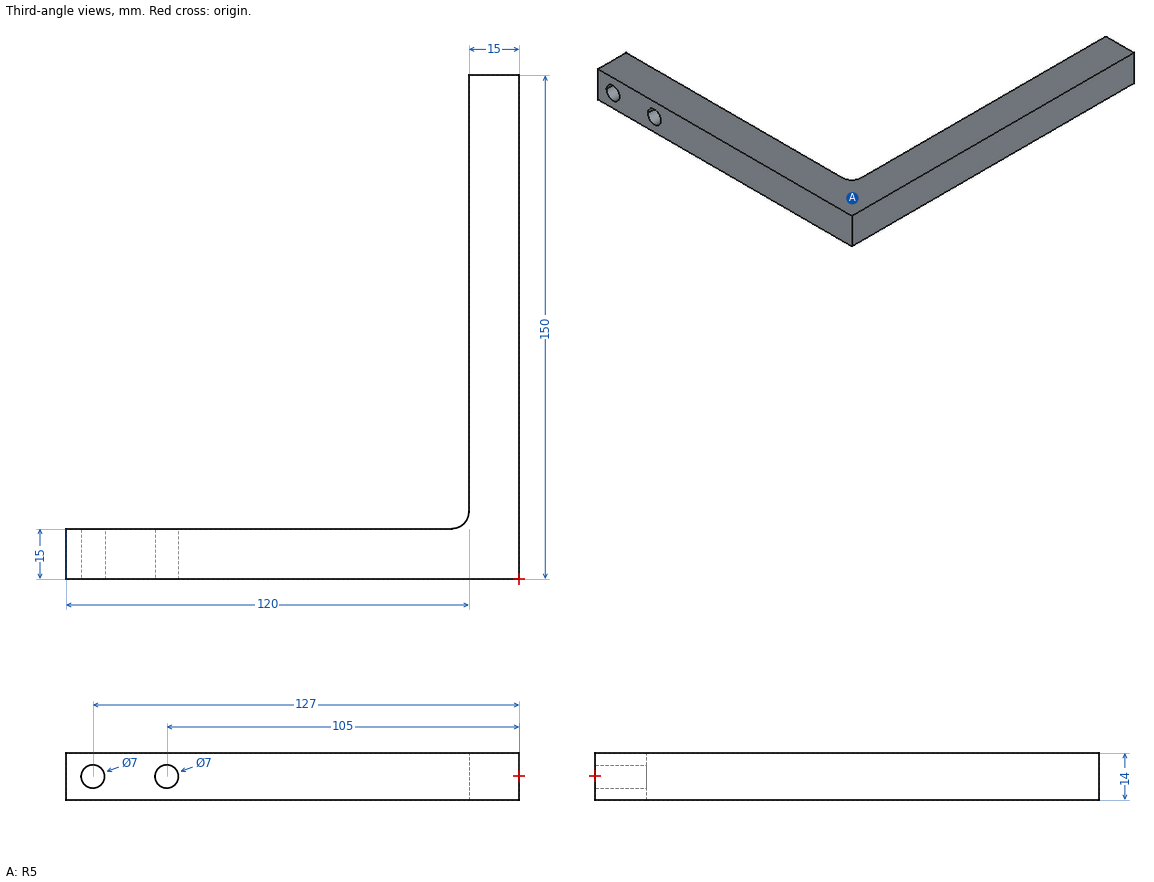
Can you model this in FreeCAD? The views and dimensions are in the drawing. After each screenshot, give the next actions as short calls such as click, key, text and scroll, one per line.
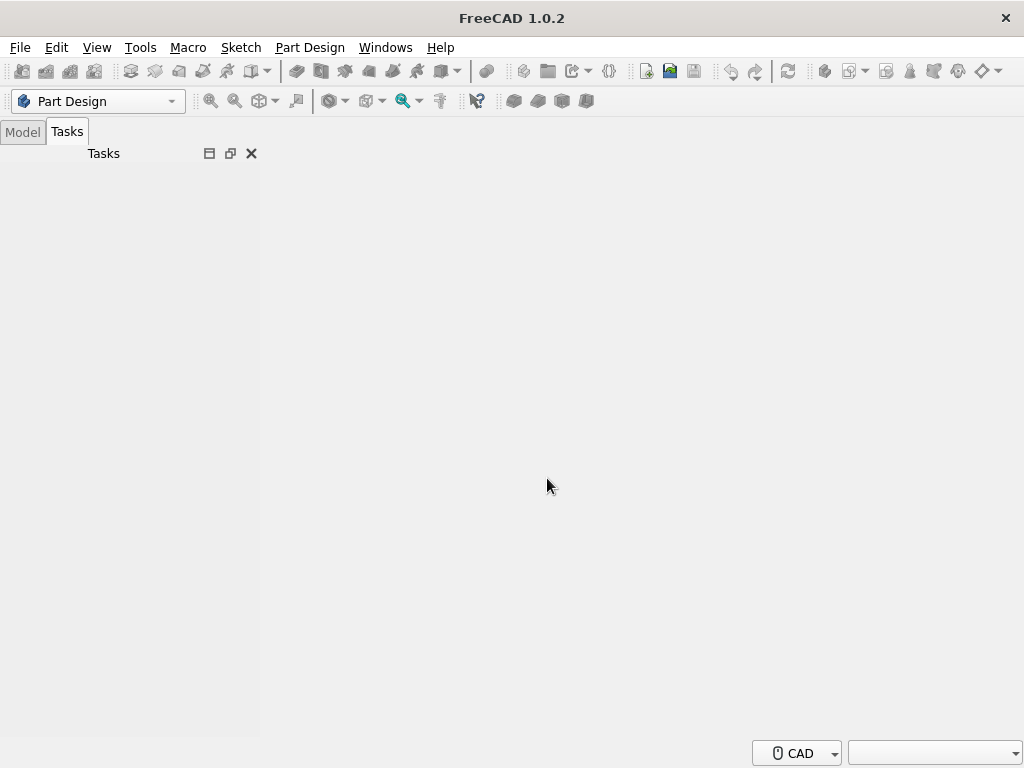
click(646, 72)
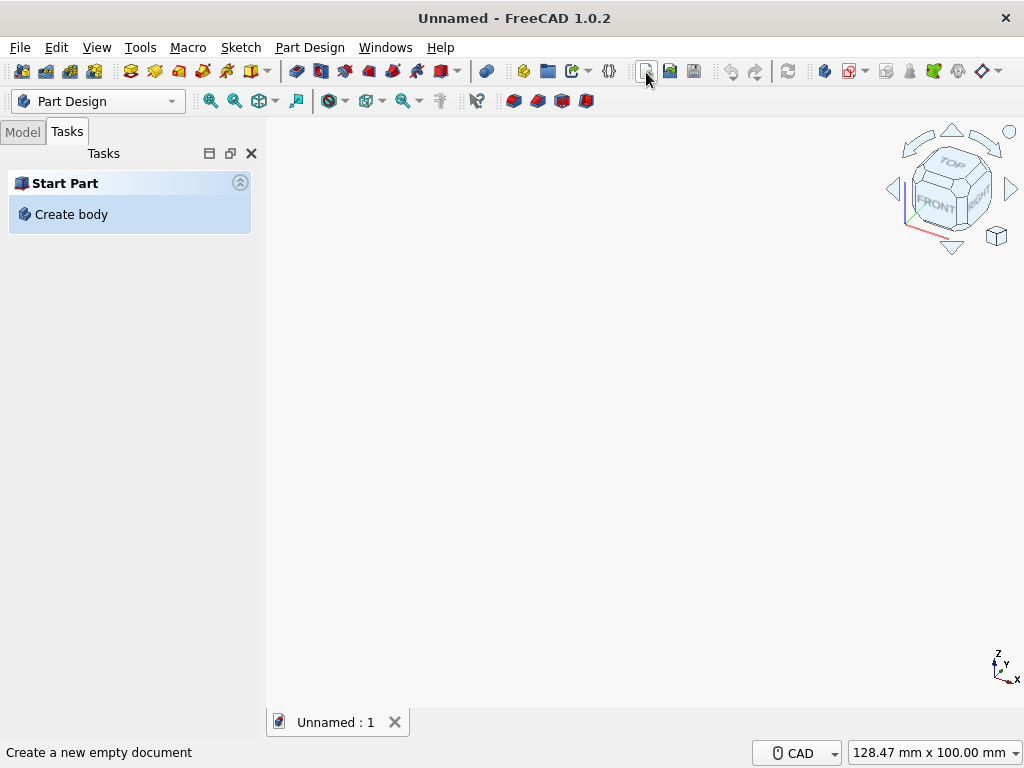
click(850, 72)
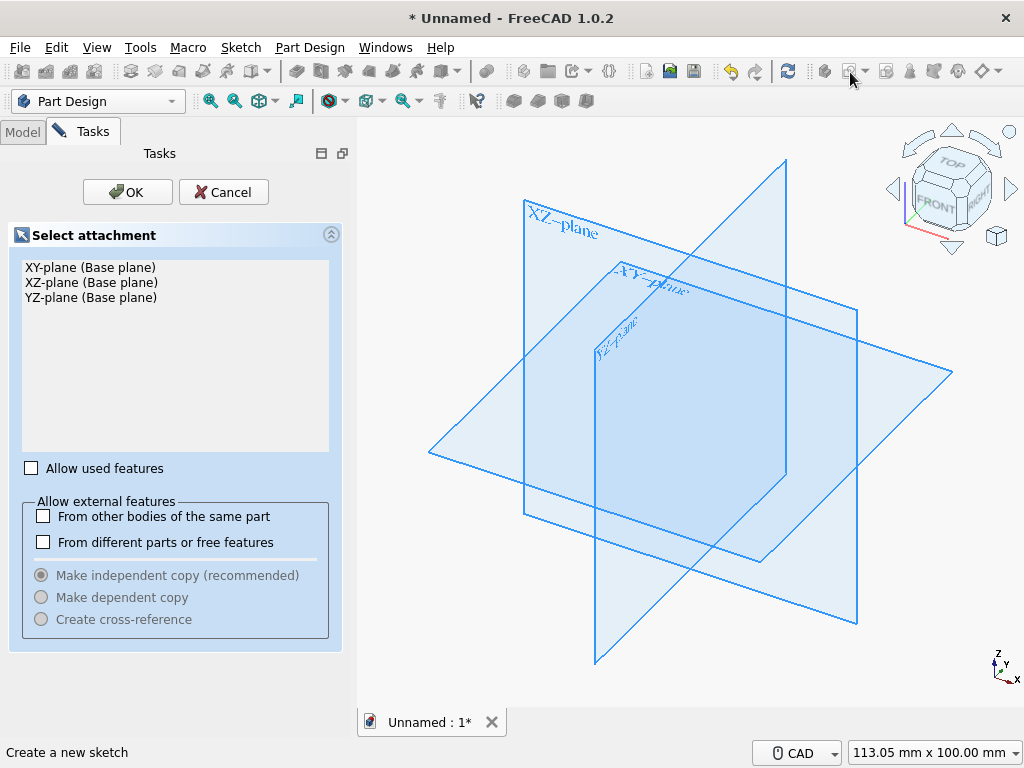
click(82, 268)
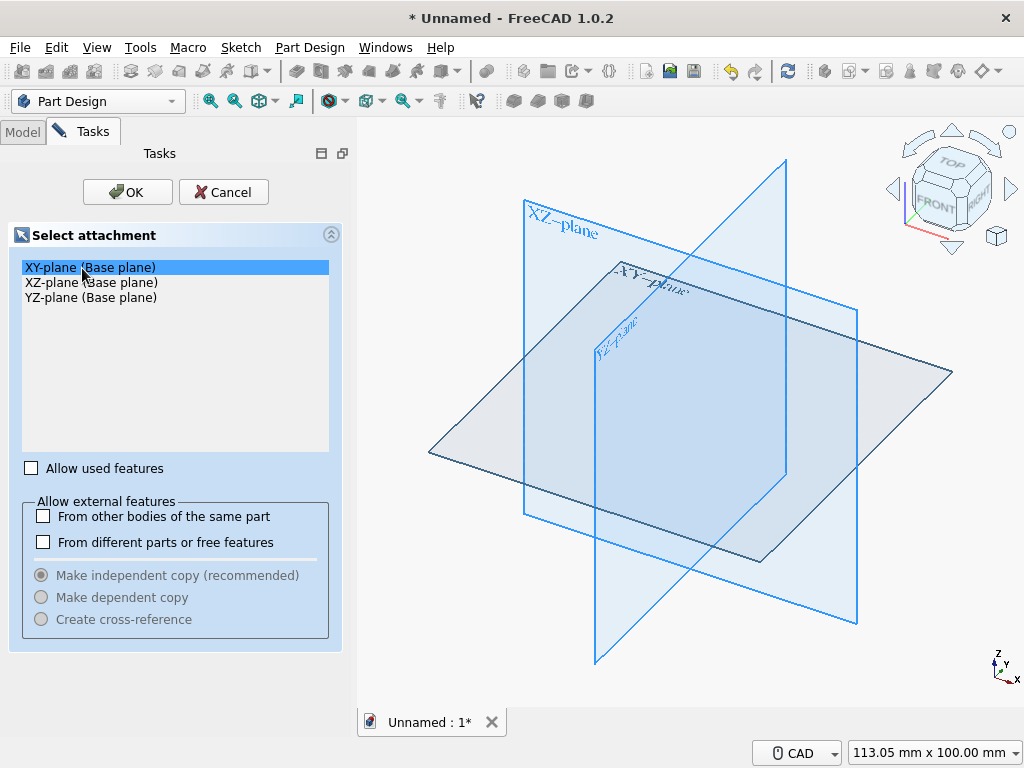
click(128, 192)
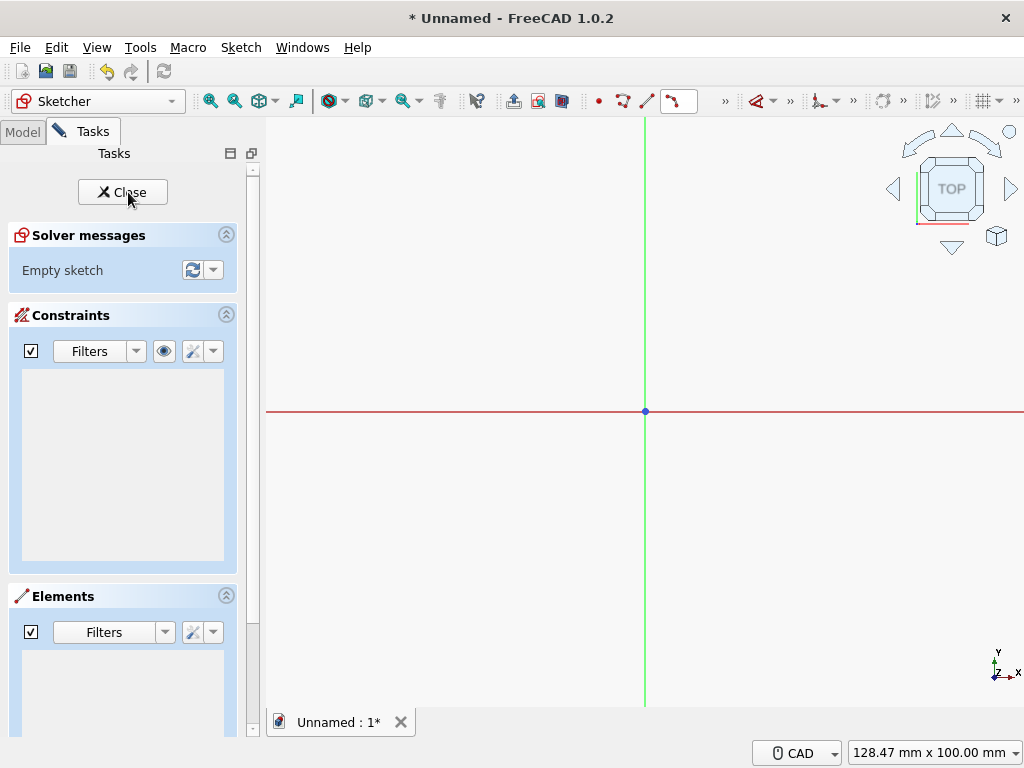
scroll(768, 670, down, 5)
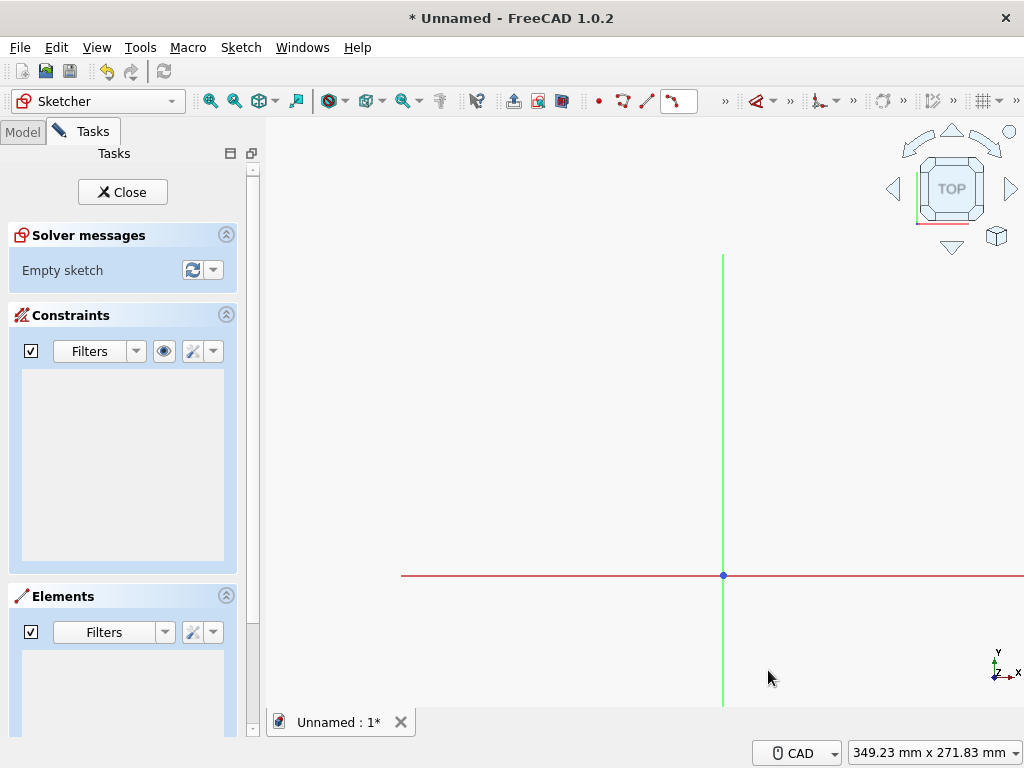
click(624, 102)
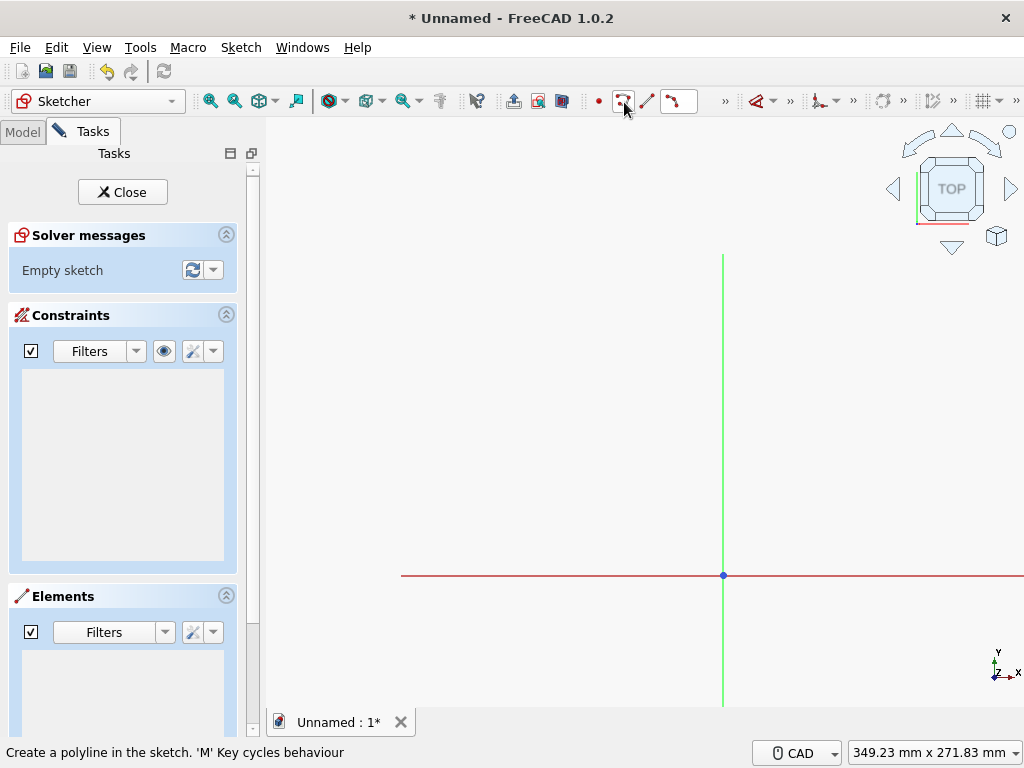
click(723, 576)
click(714, 250)
click(691, 250)
click(691, 543)
click(430, 543)
click(430, 567)
click(723, 576)
key(Escape)
key(Escape)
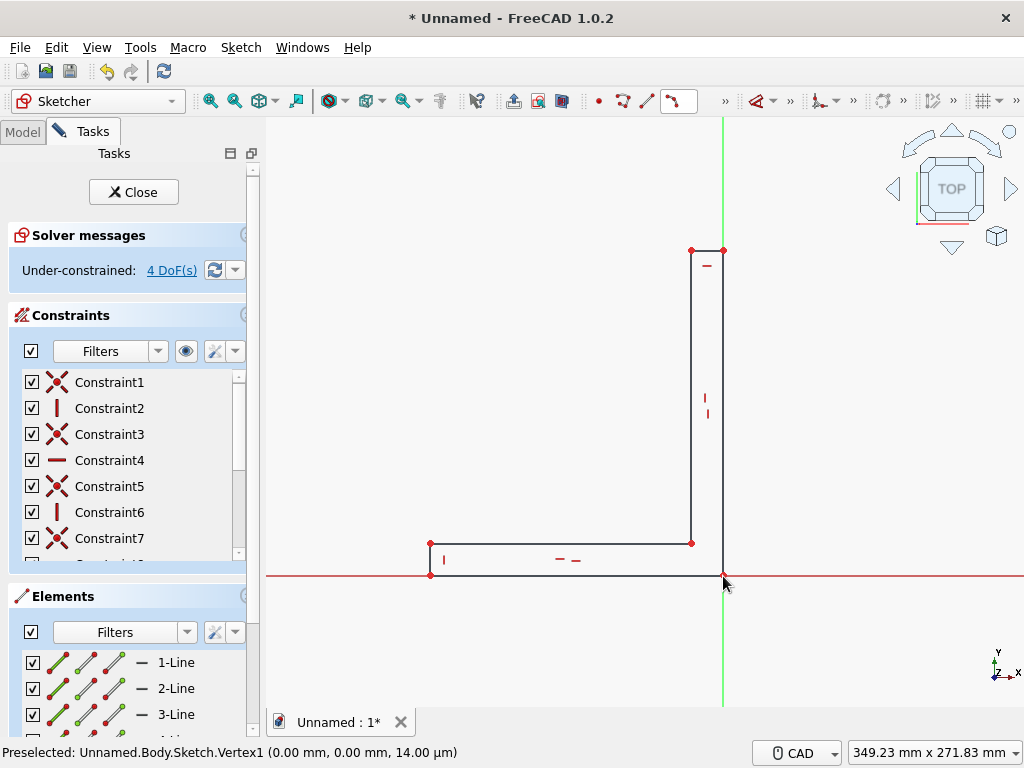
key(d)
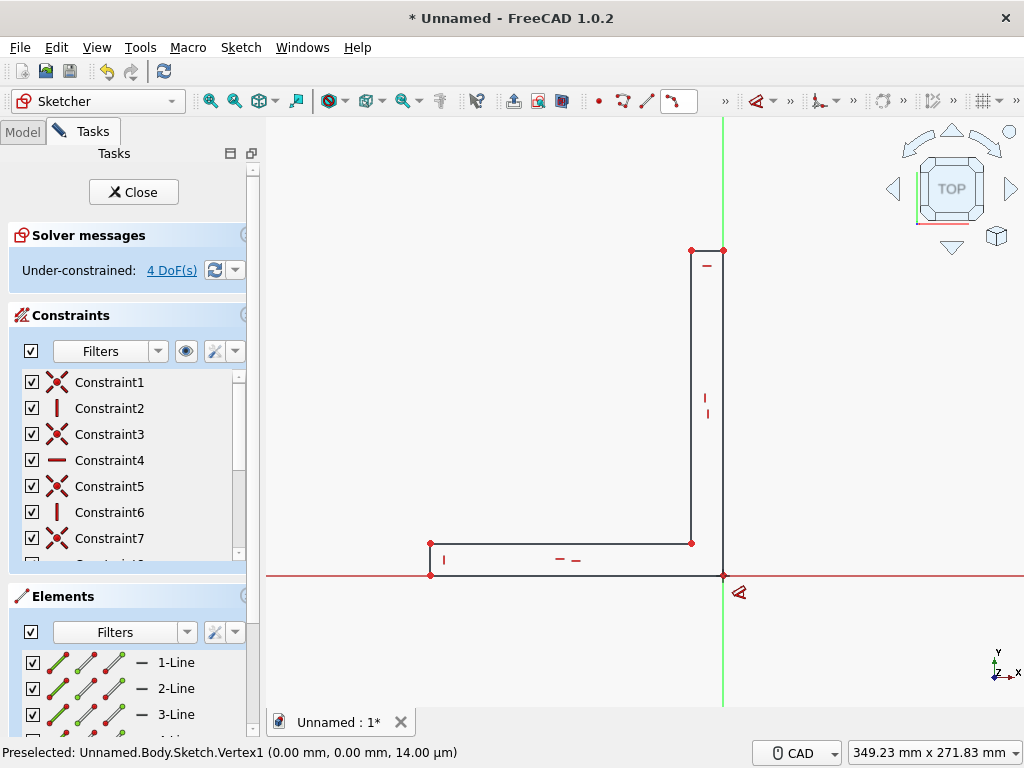
scroll(714, 251, up, 2)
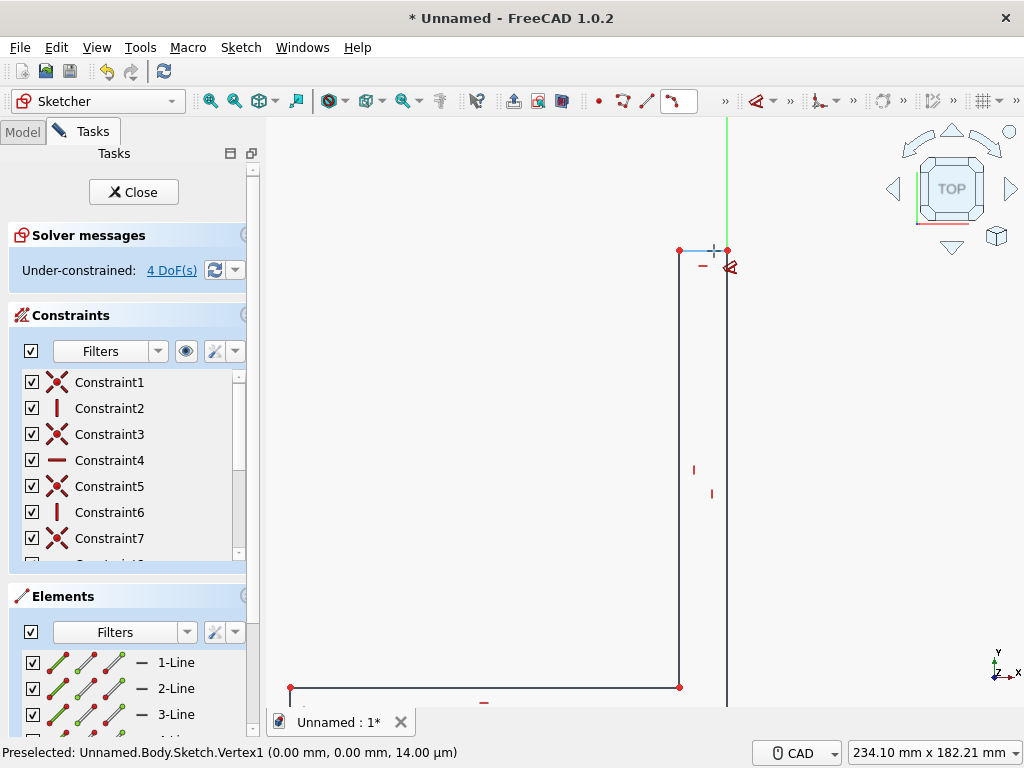
click(713, 251)
click(703, 217)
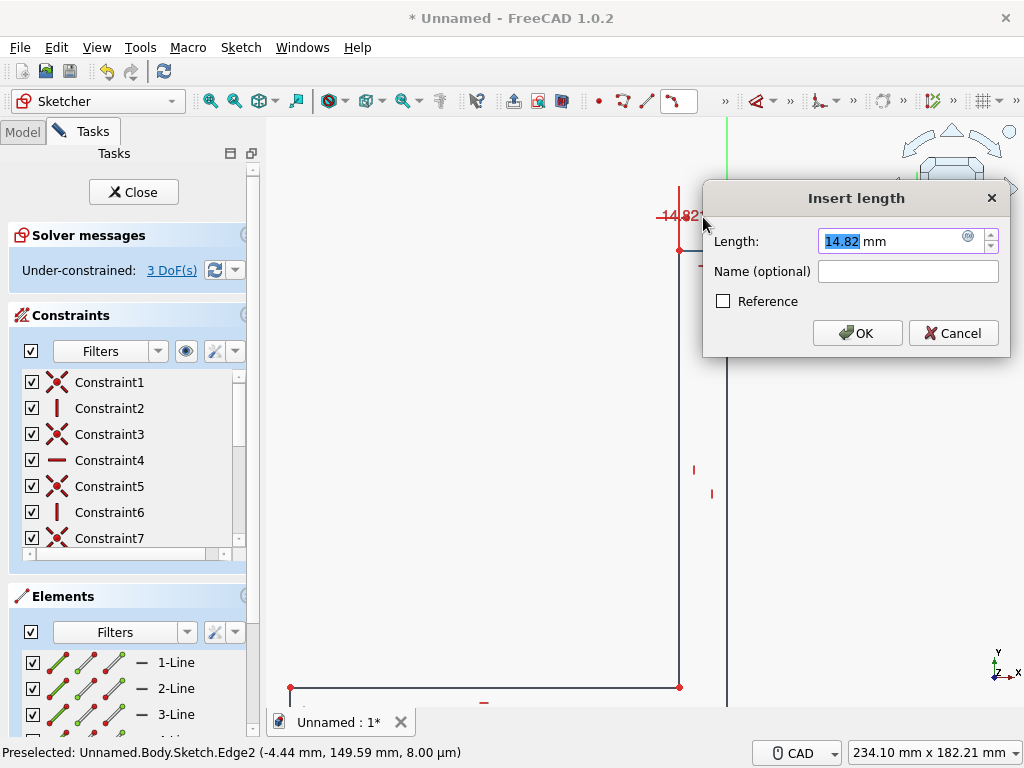
text(15)
key(Return)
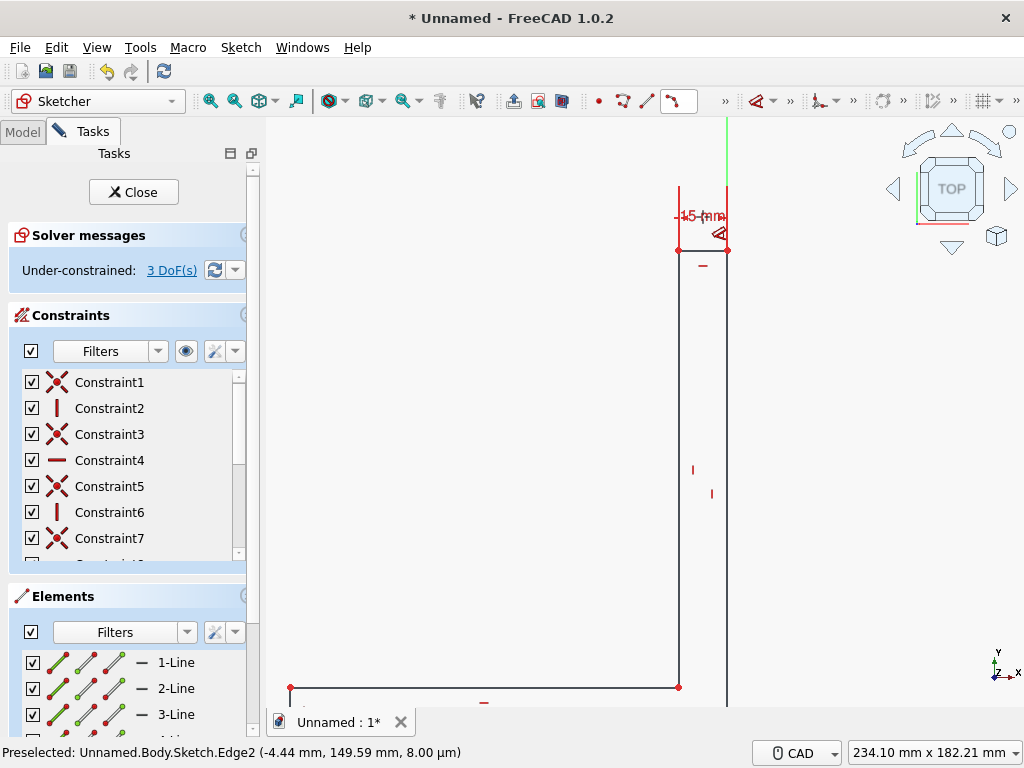
scroll(859, 145, down, 1)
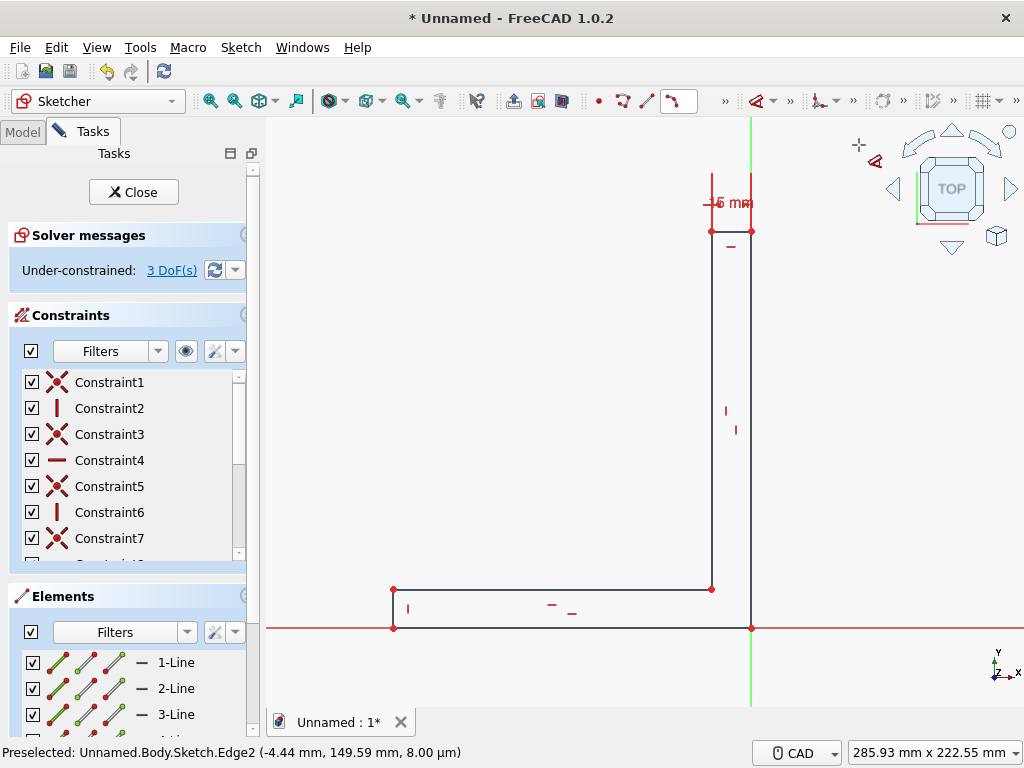
click(393, 601)
click(359, 609)